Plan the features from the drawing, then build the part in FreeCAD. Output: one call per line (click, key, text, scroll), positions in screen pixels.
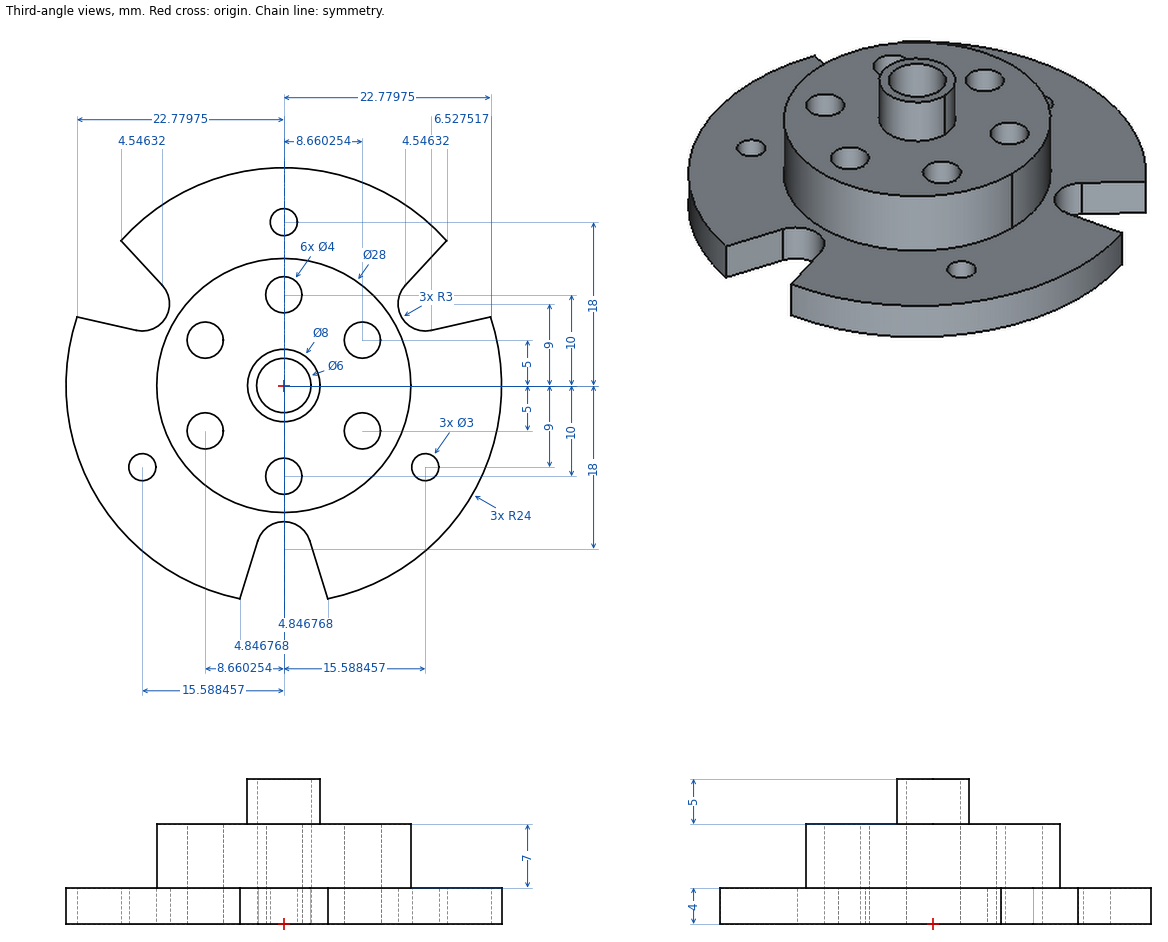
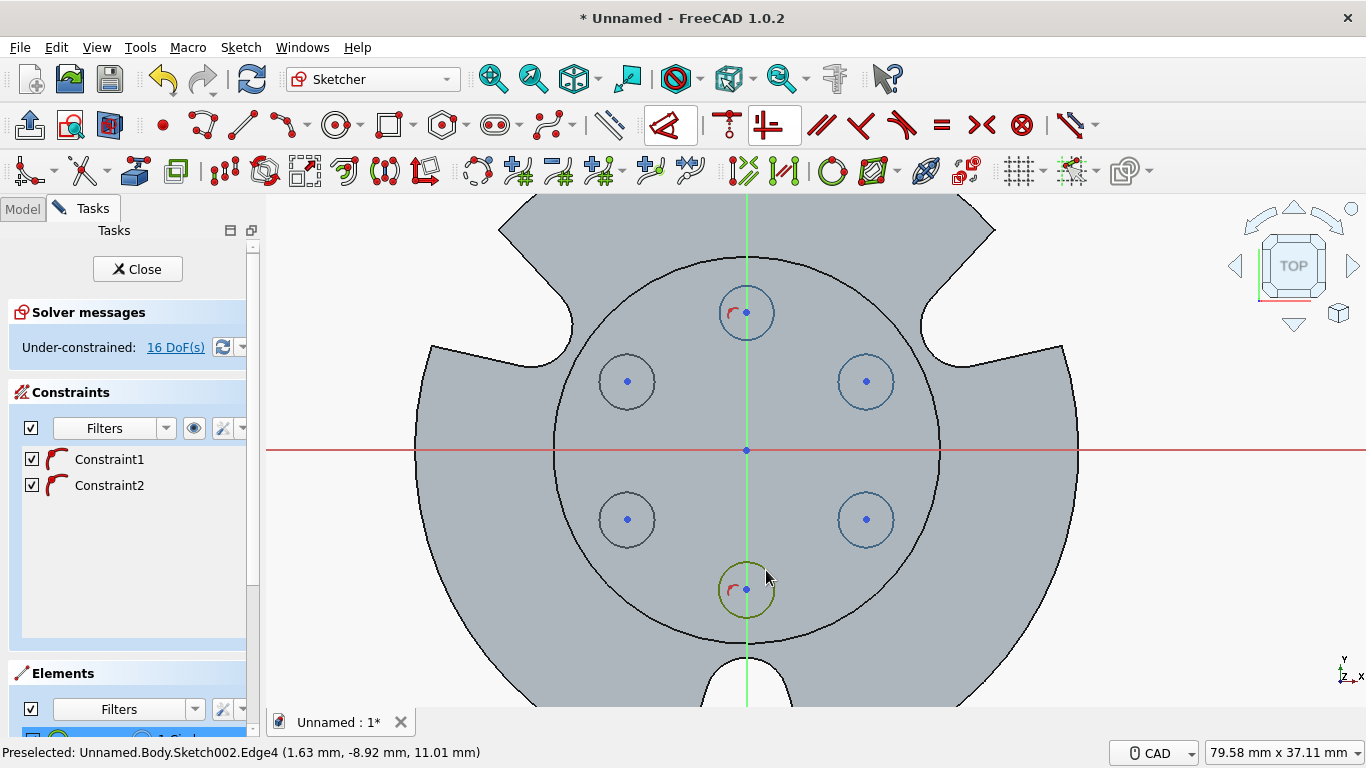
click(646, 500)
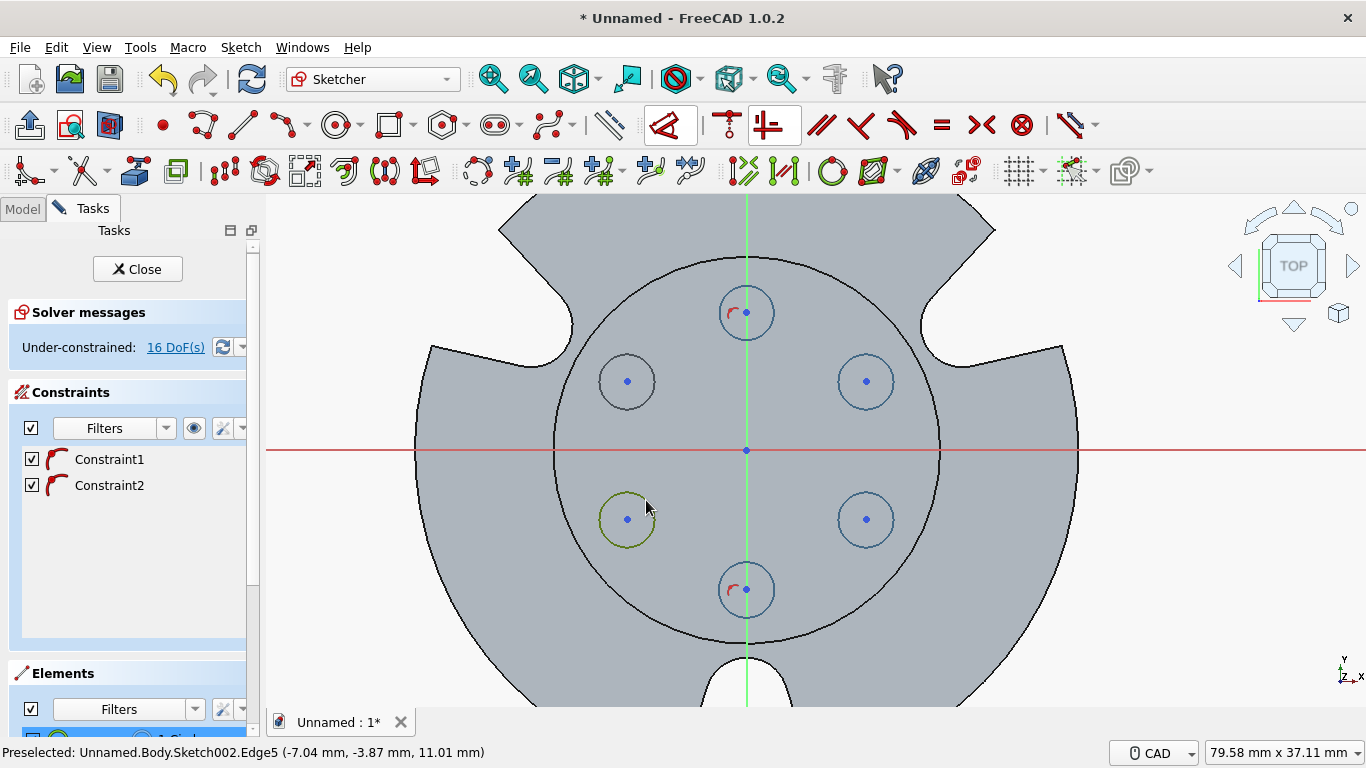
click(646, 362)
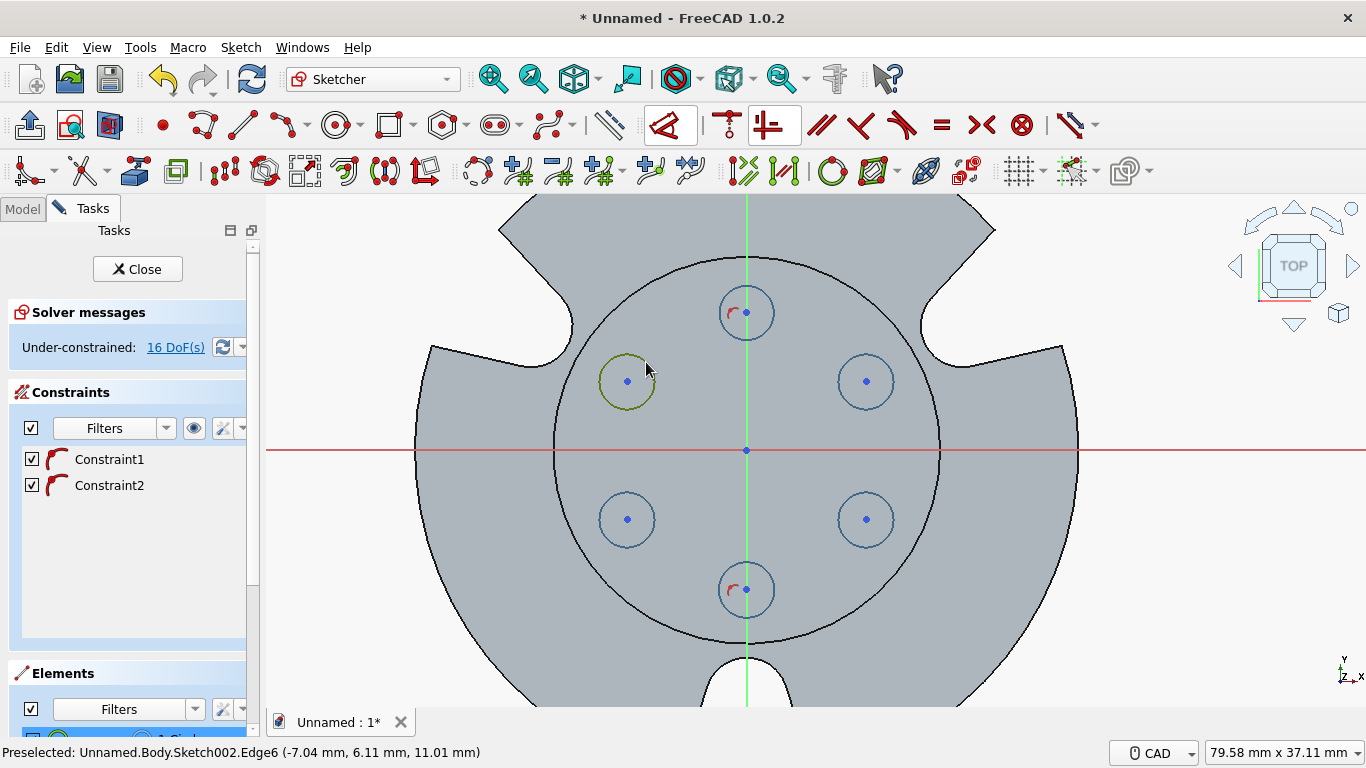
key(e)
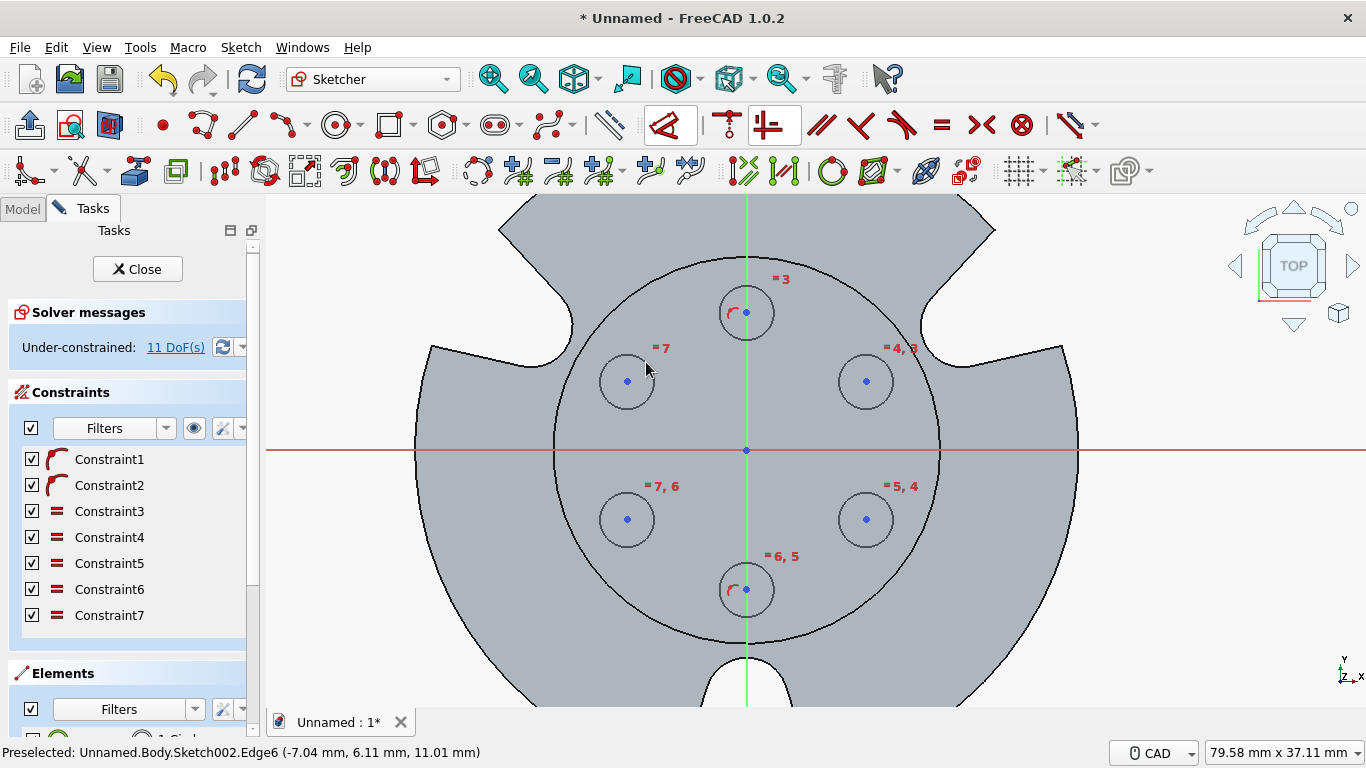
click(866, 382)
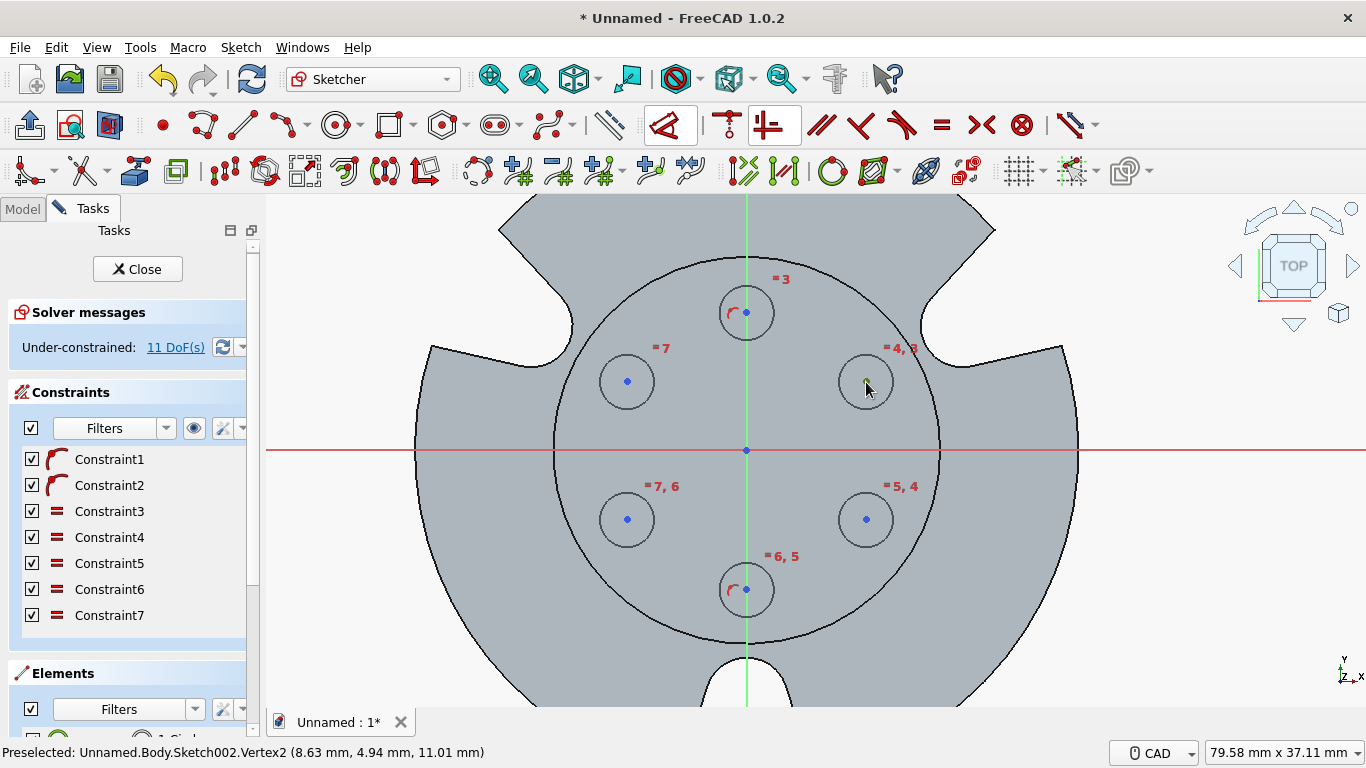
click(866, 520)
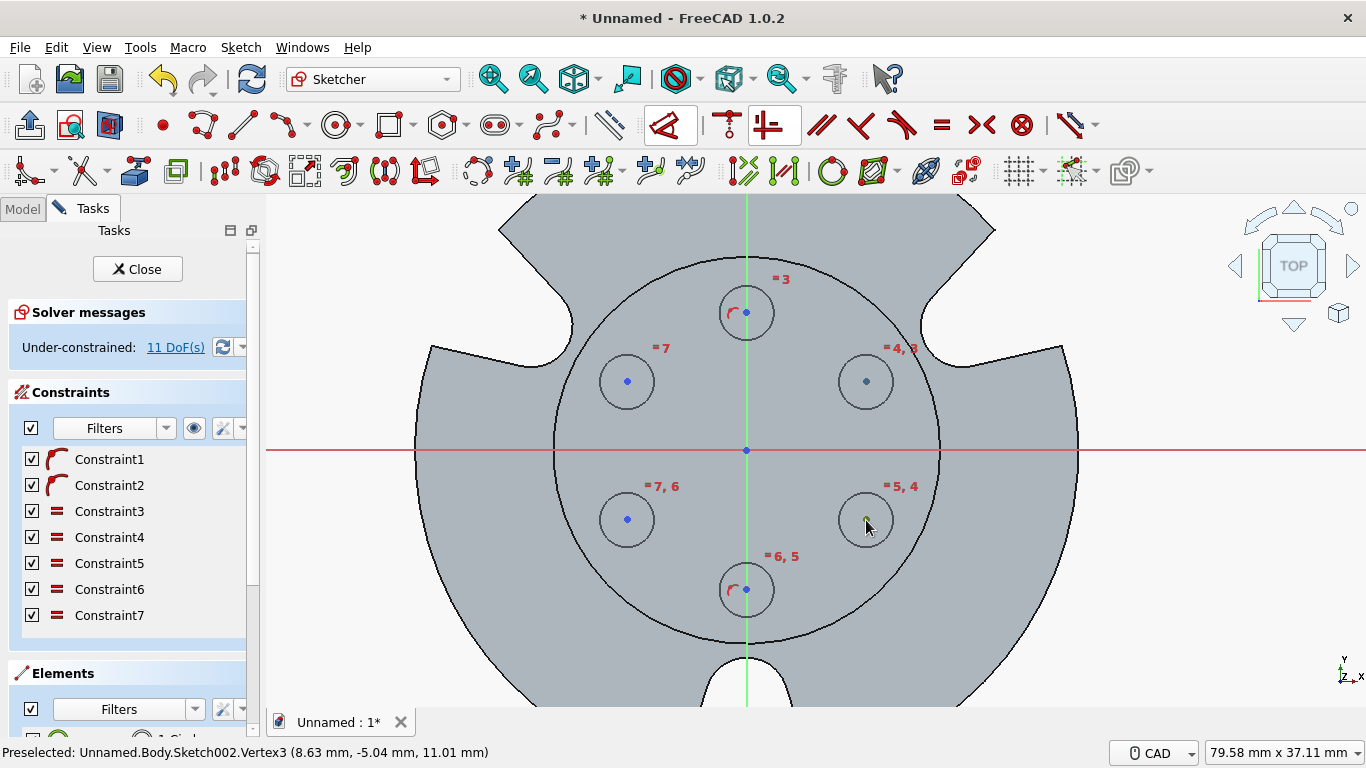
key(v)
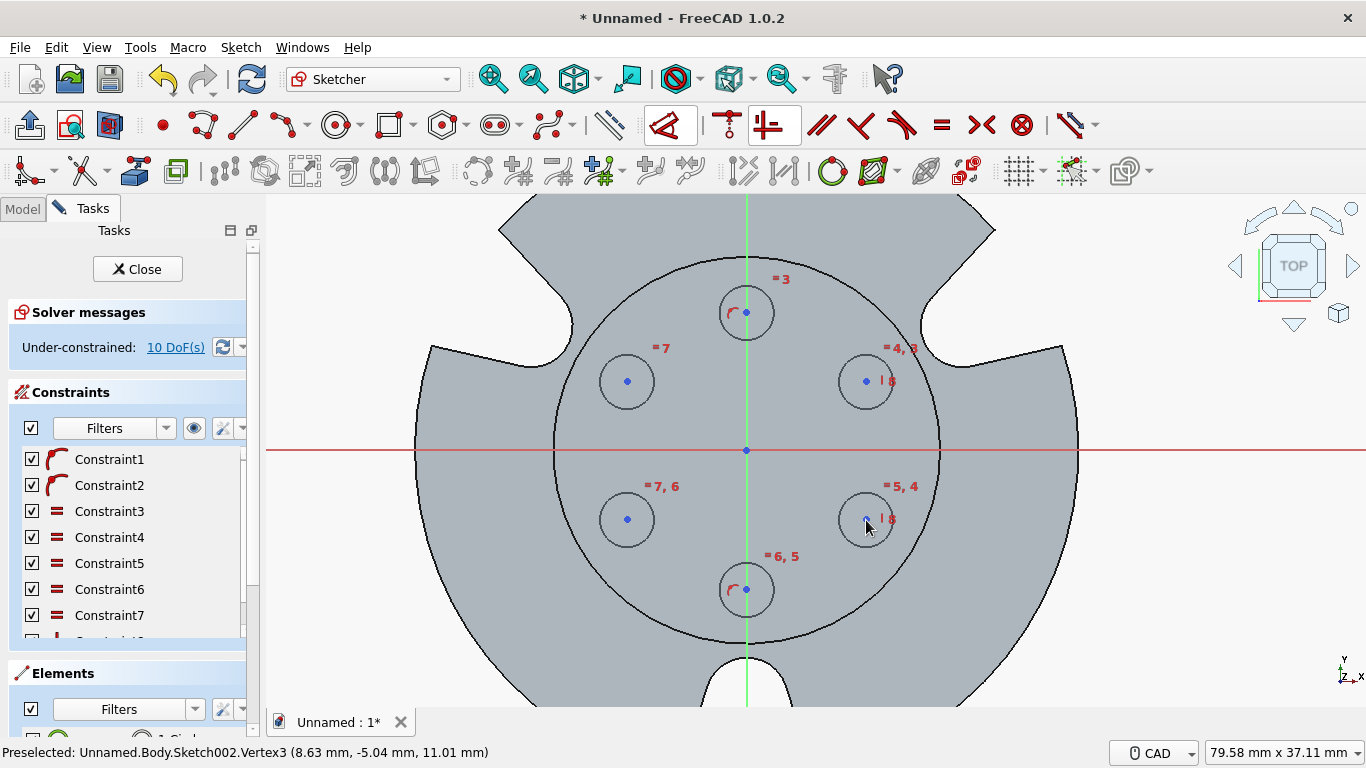
click(866, 520)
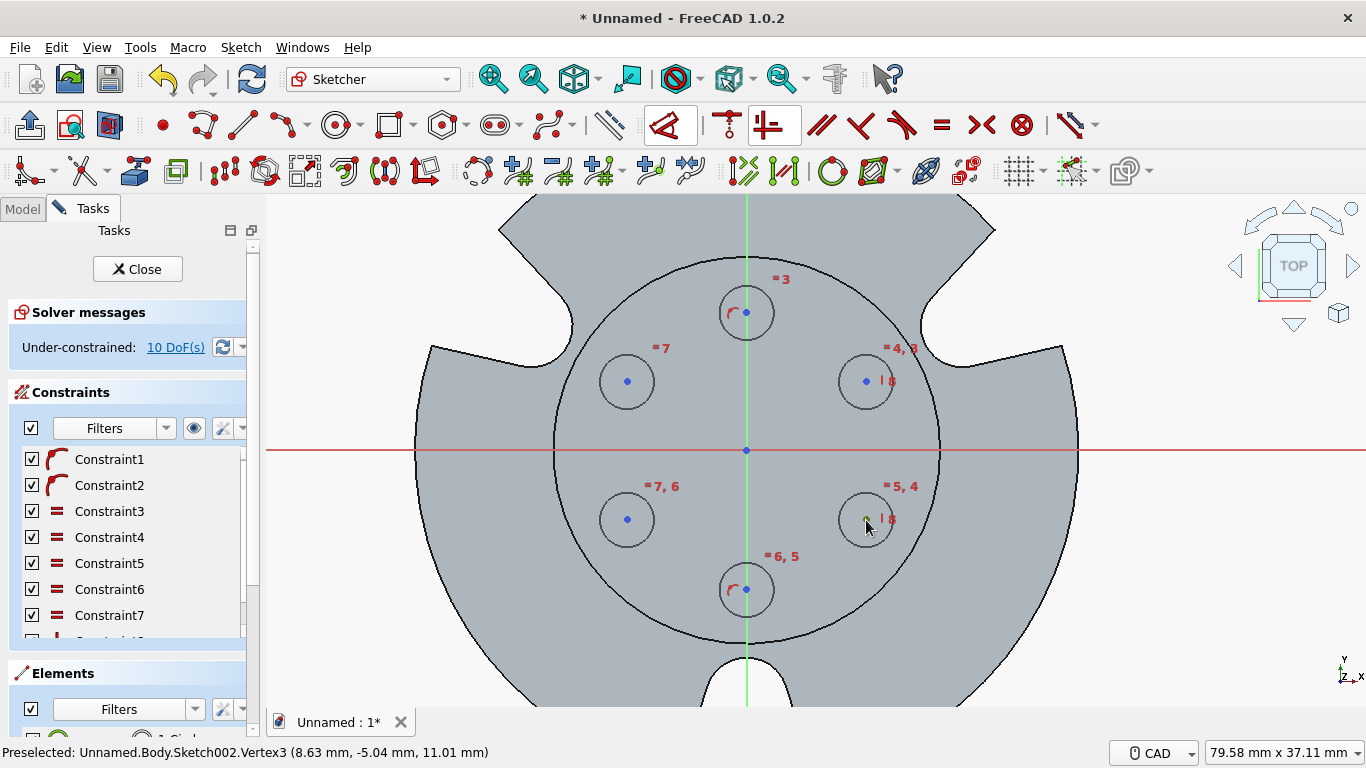
click(627, 520)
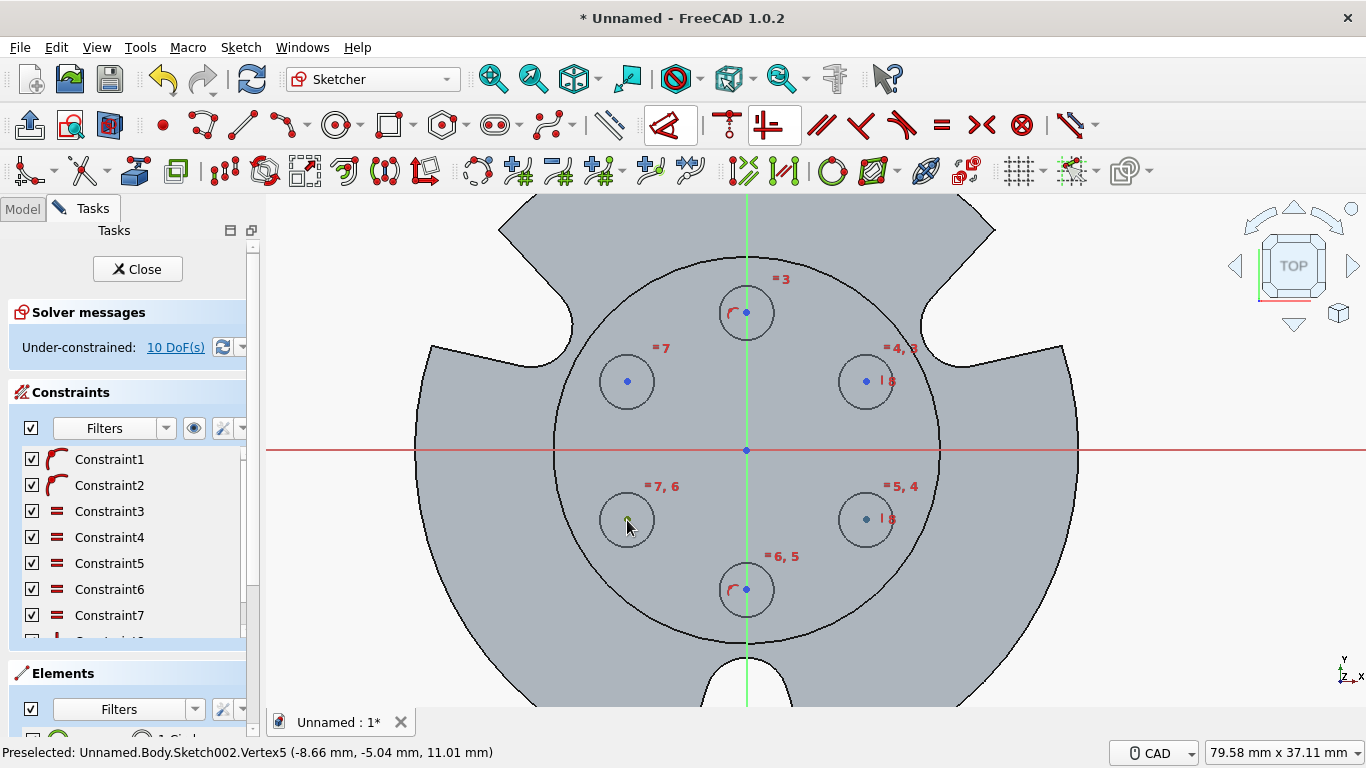
click(796, 126)